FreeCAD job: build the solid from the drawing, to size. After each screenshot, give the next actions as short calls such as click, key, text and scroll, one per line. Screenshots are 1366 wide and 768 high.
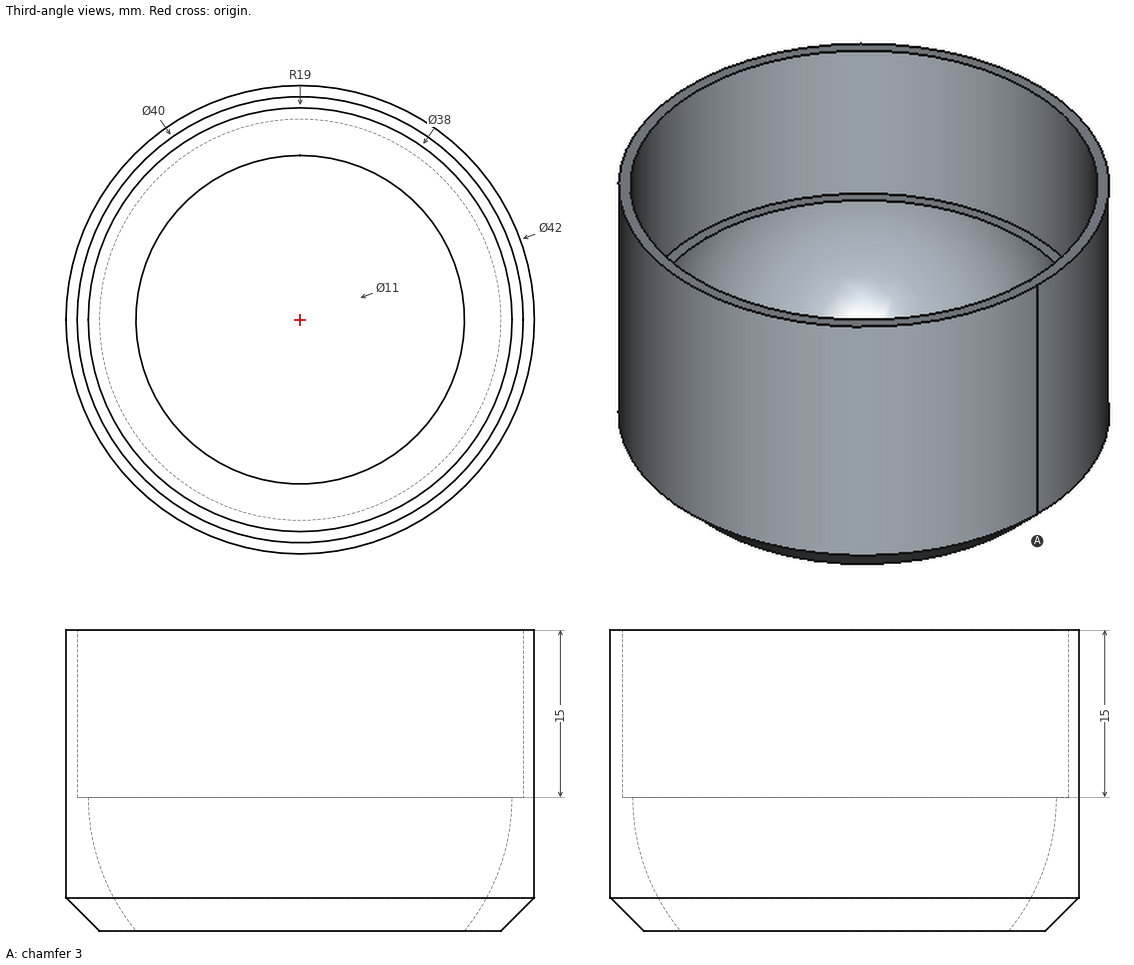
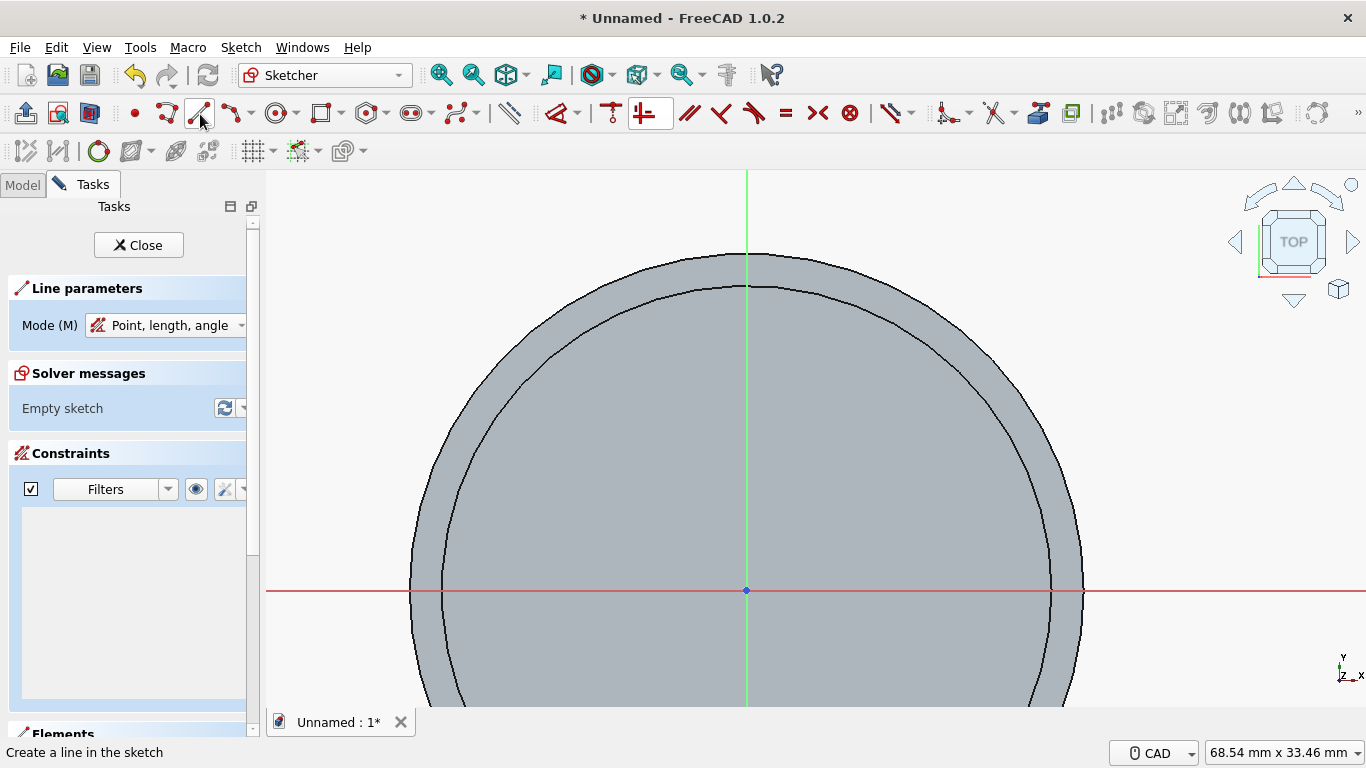
click(442, 591)
click(1052, 582)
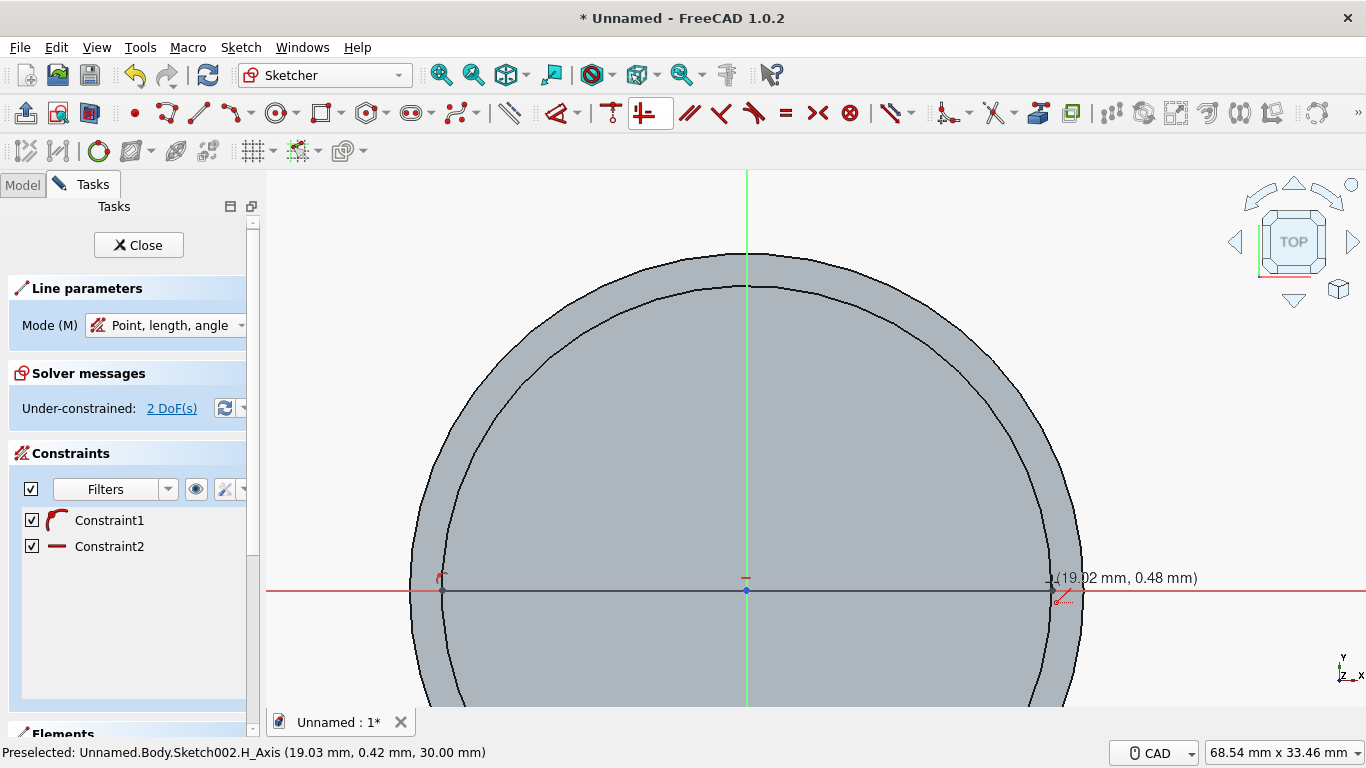
click(232, 114)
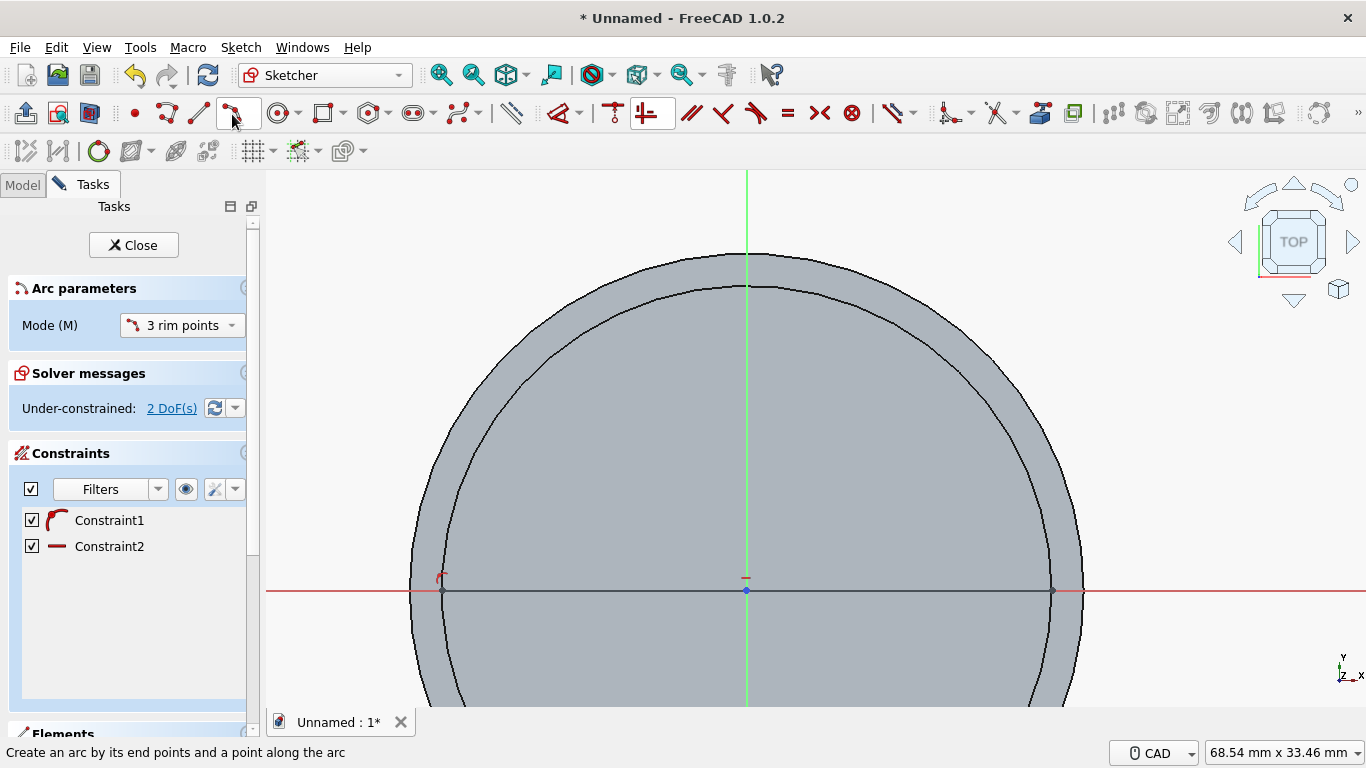
click(1052, 591)
click(442, 591)
click(841, 301)
key(Escape)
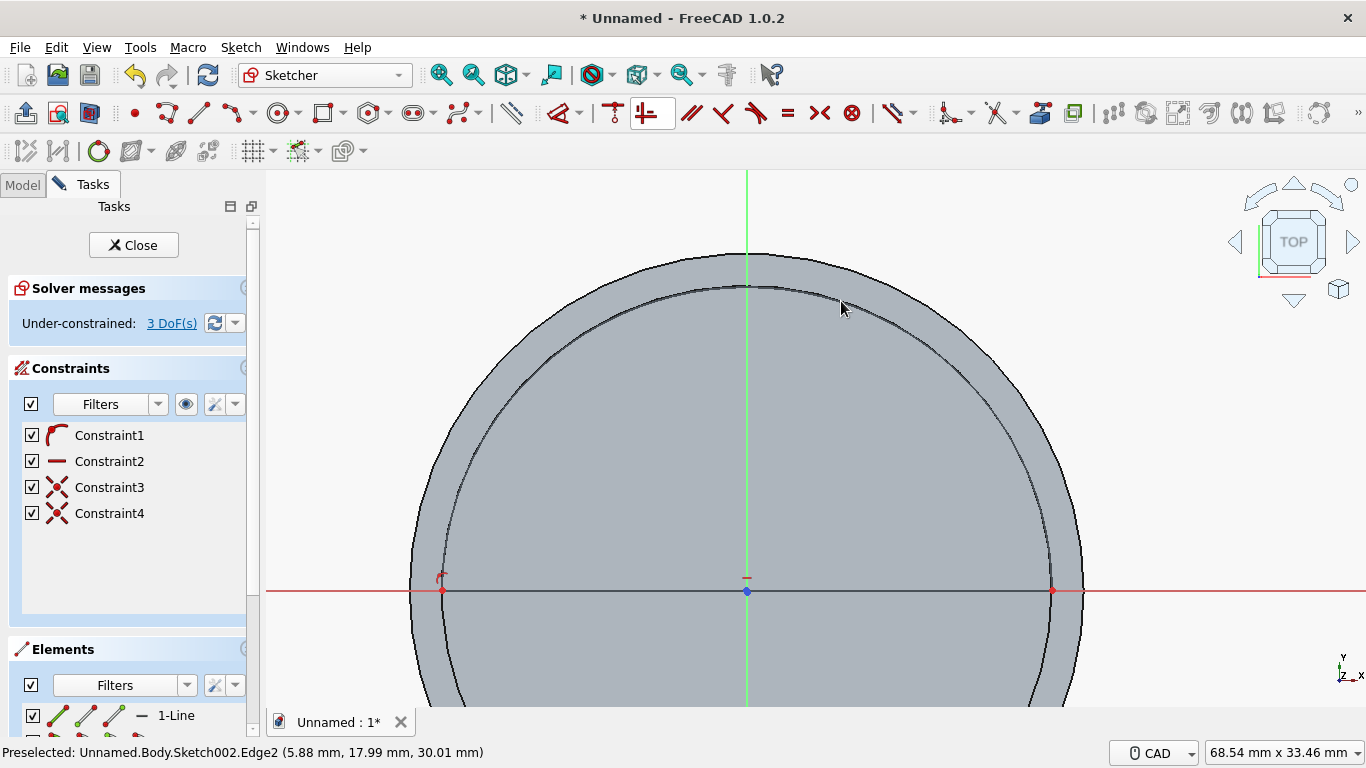
drag(737, 581, 757, 602)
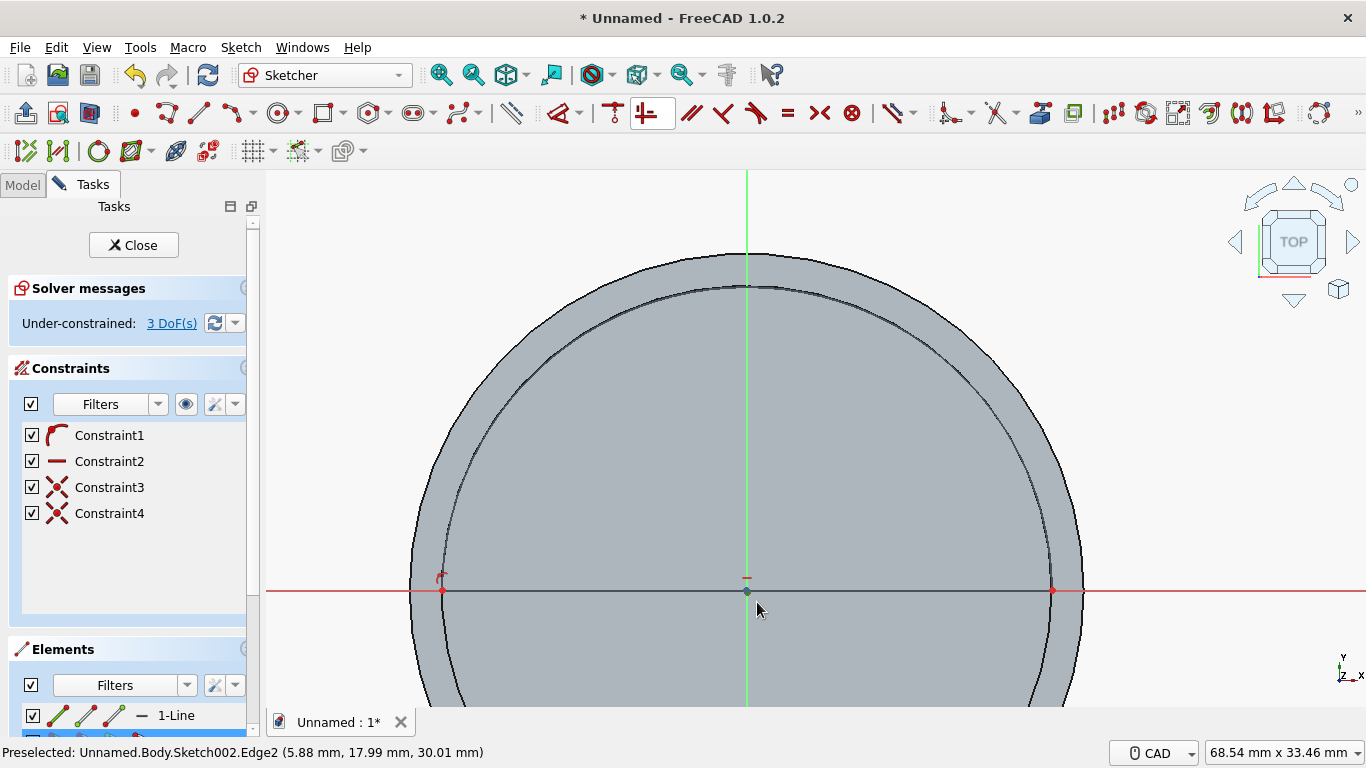
click(614, 114)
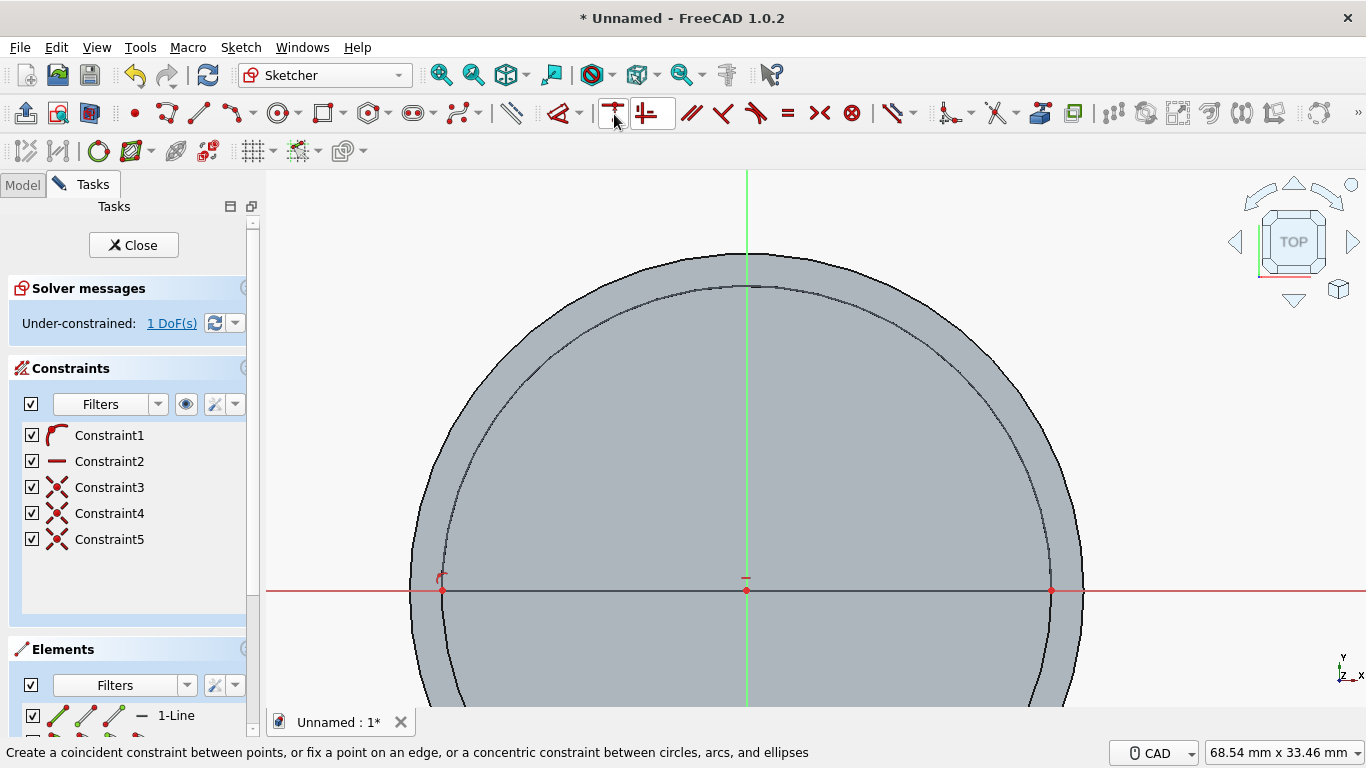
click(558, 114)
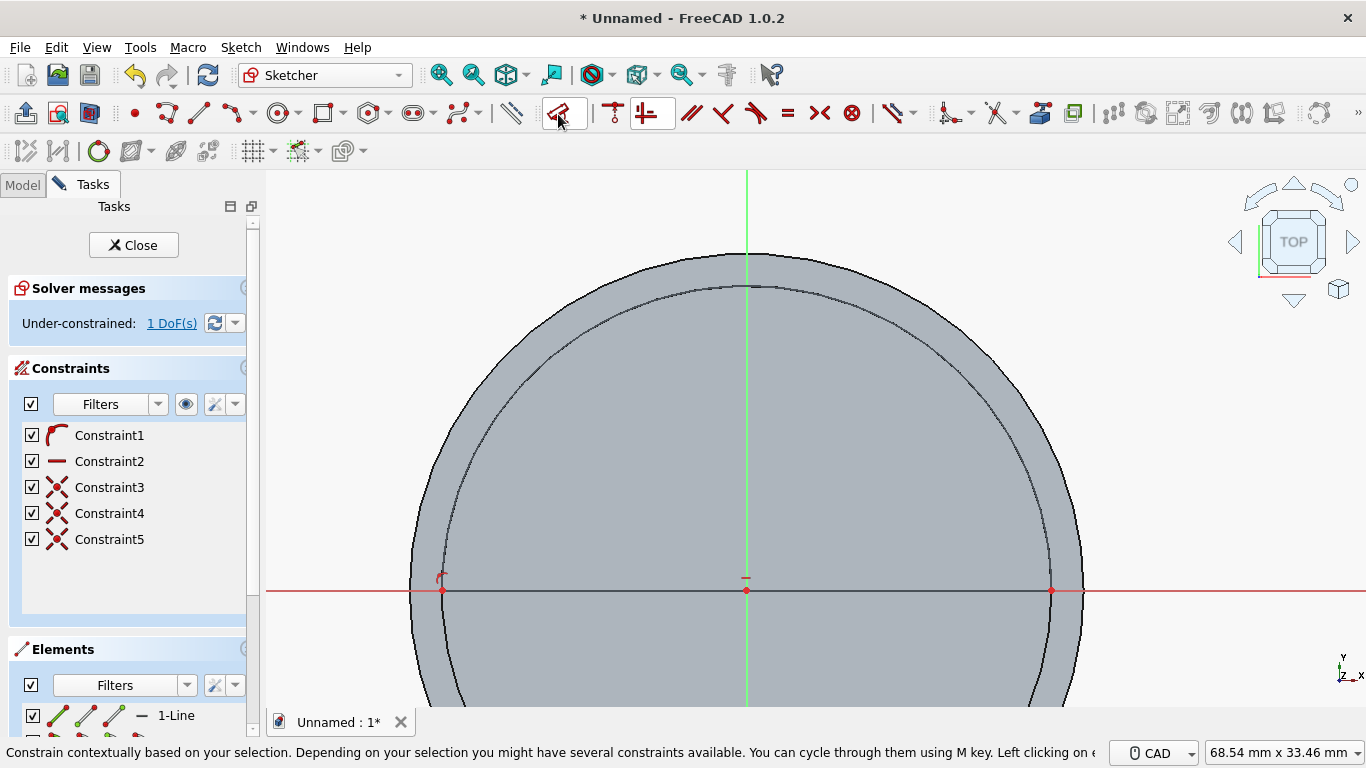
click(926, 344)
click(945, 318)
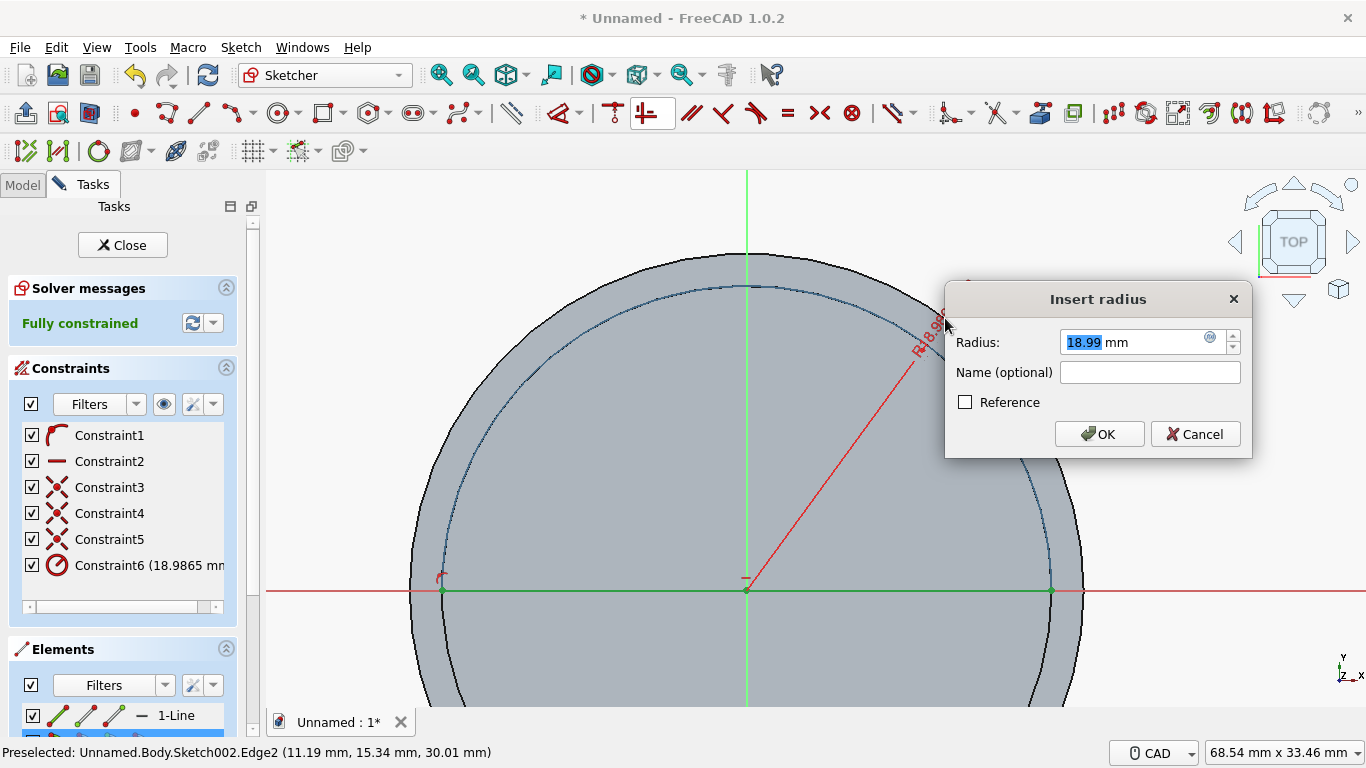
text(19)
key(Return)
key(Escape)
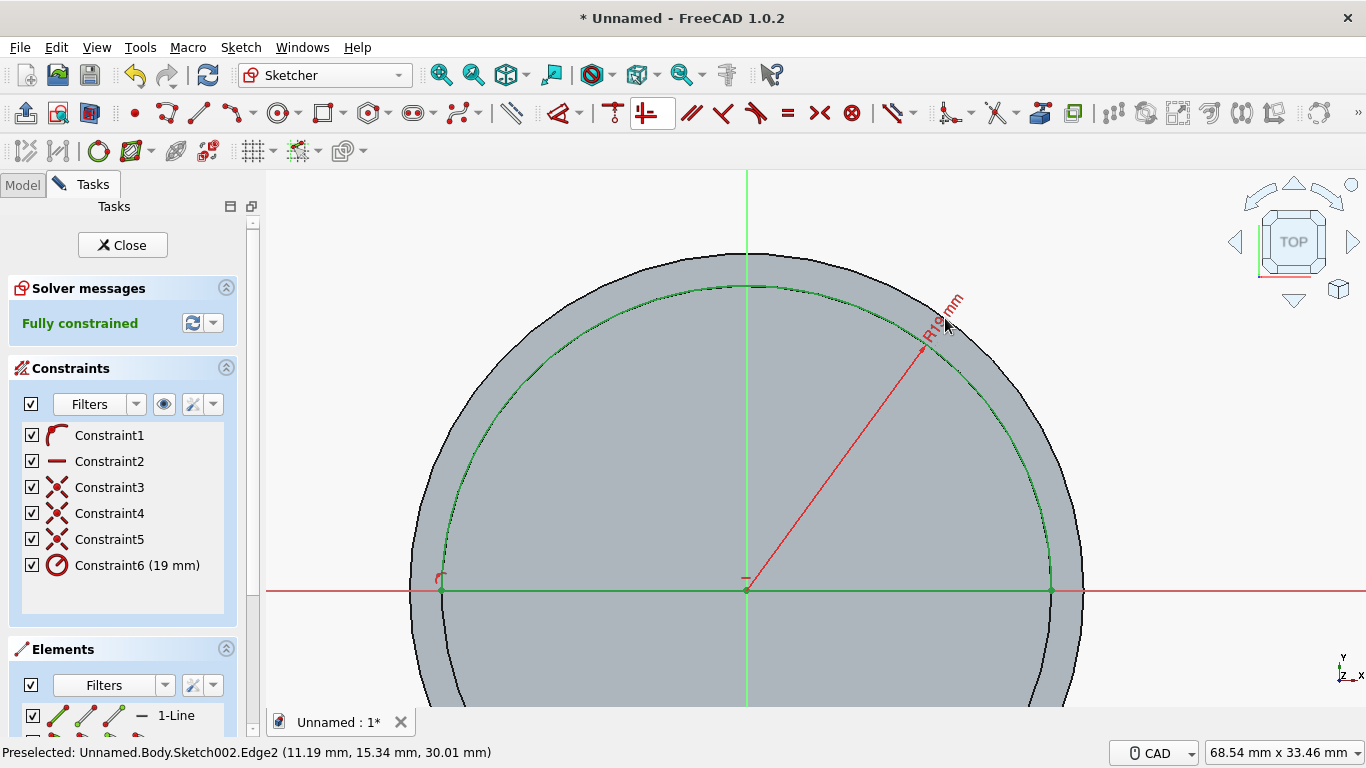
click(123, 245)